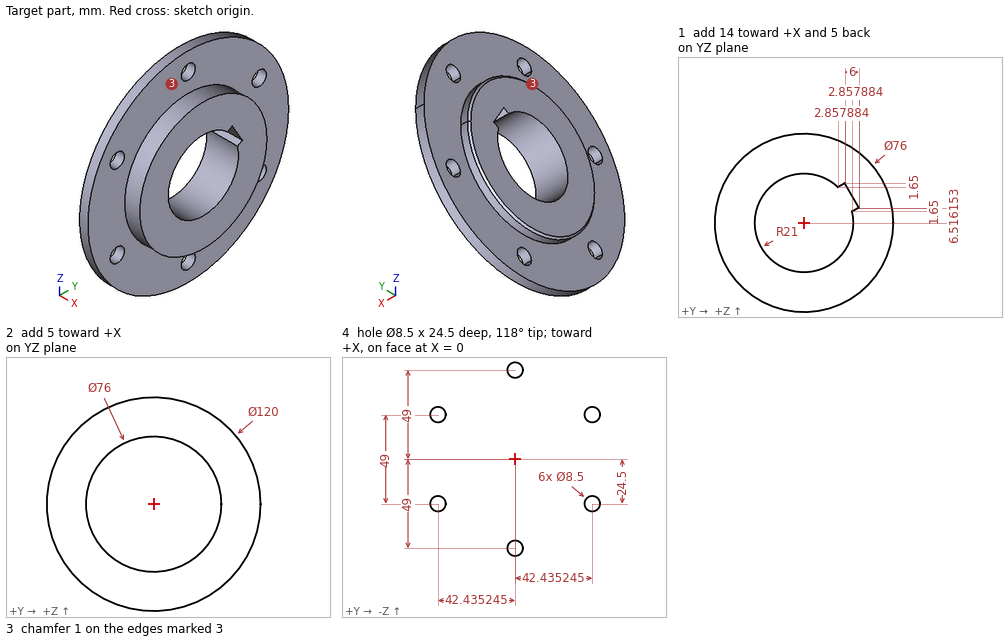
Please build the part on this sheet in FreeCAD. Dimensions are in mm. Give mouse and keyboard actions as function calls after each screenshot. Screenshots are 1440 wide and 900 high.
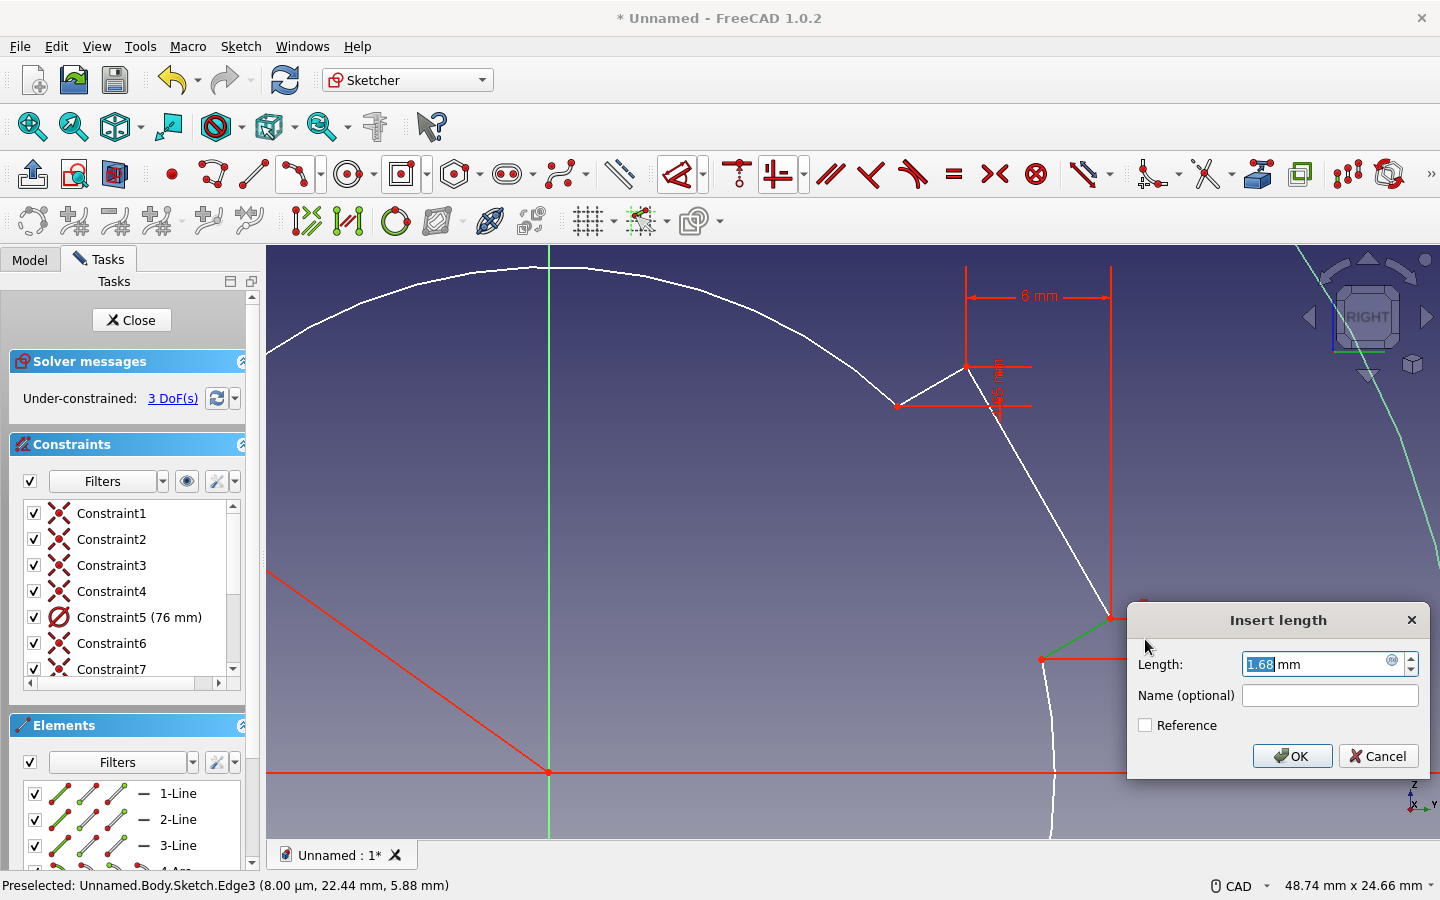
text(1.65)
key(Return)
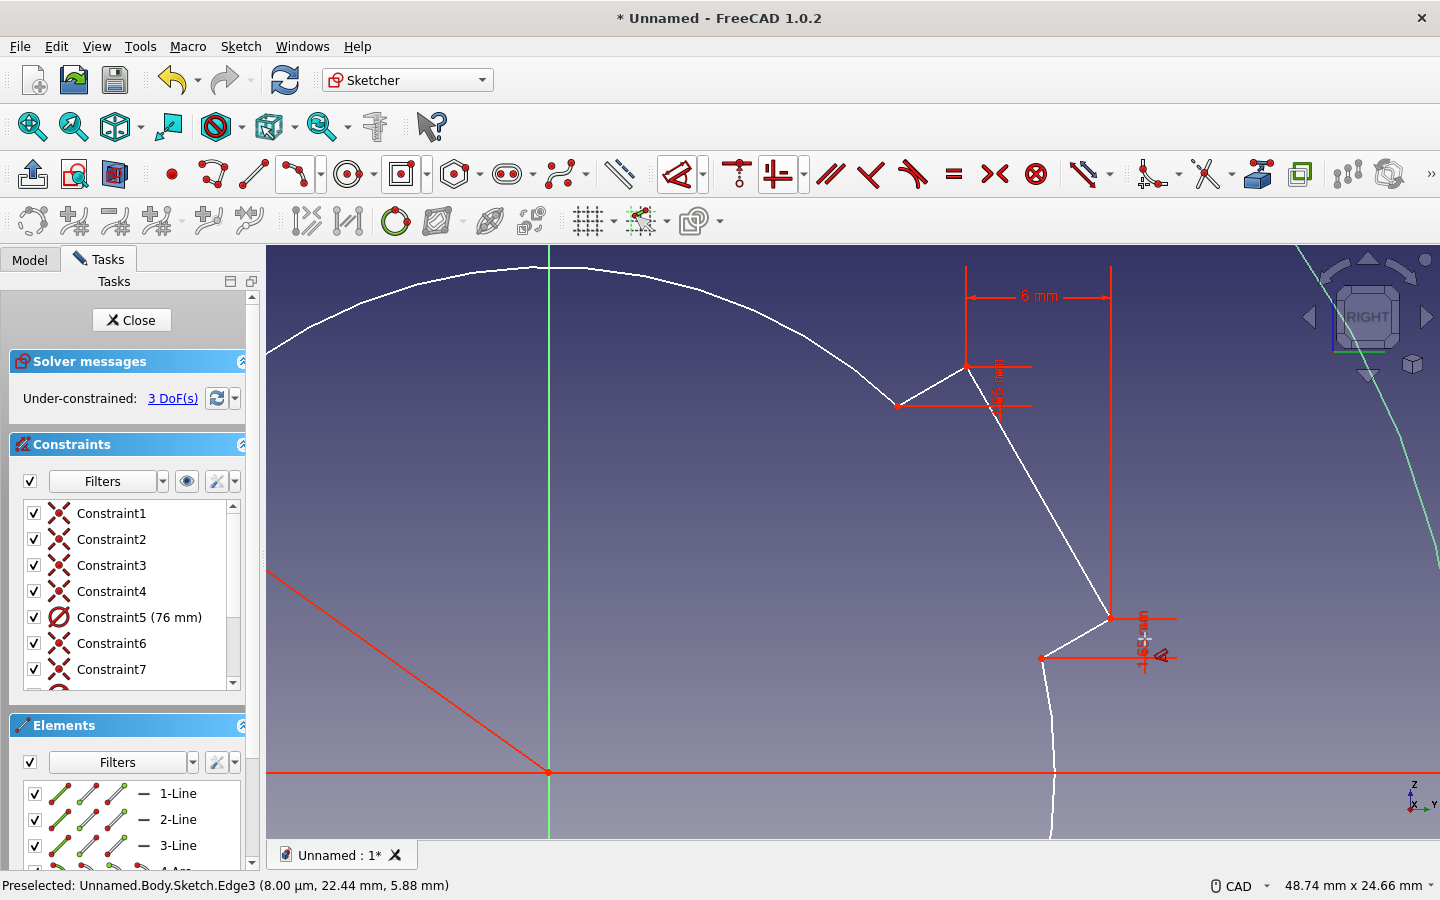
scroll(844, 484, down, 8)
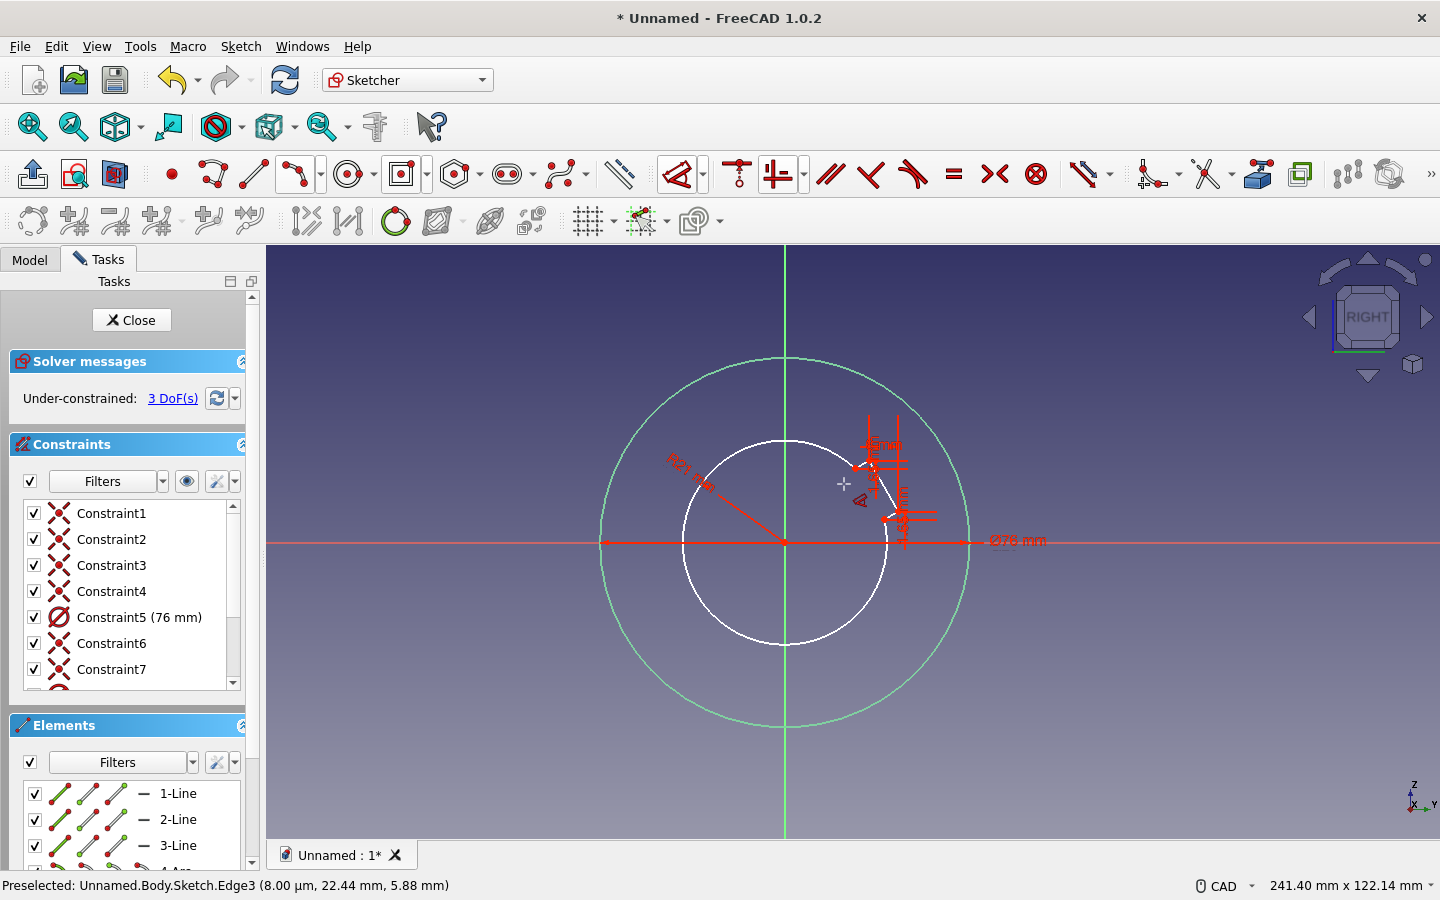
scroll(898, 512, up, 2)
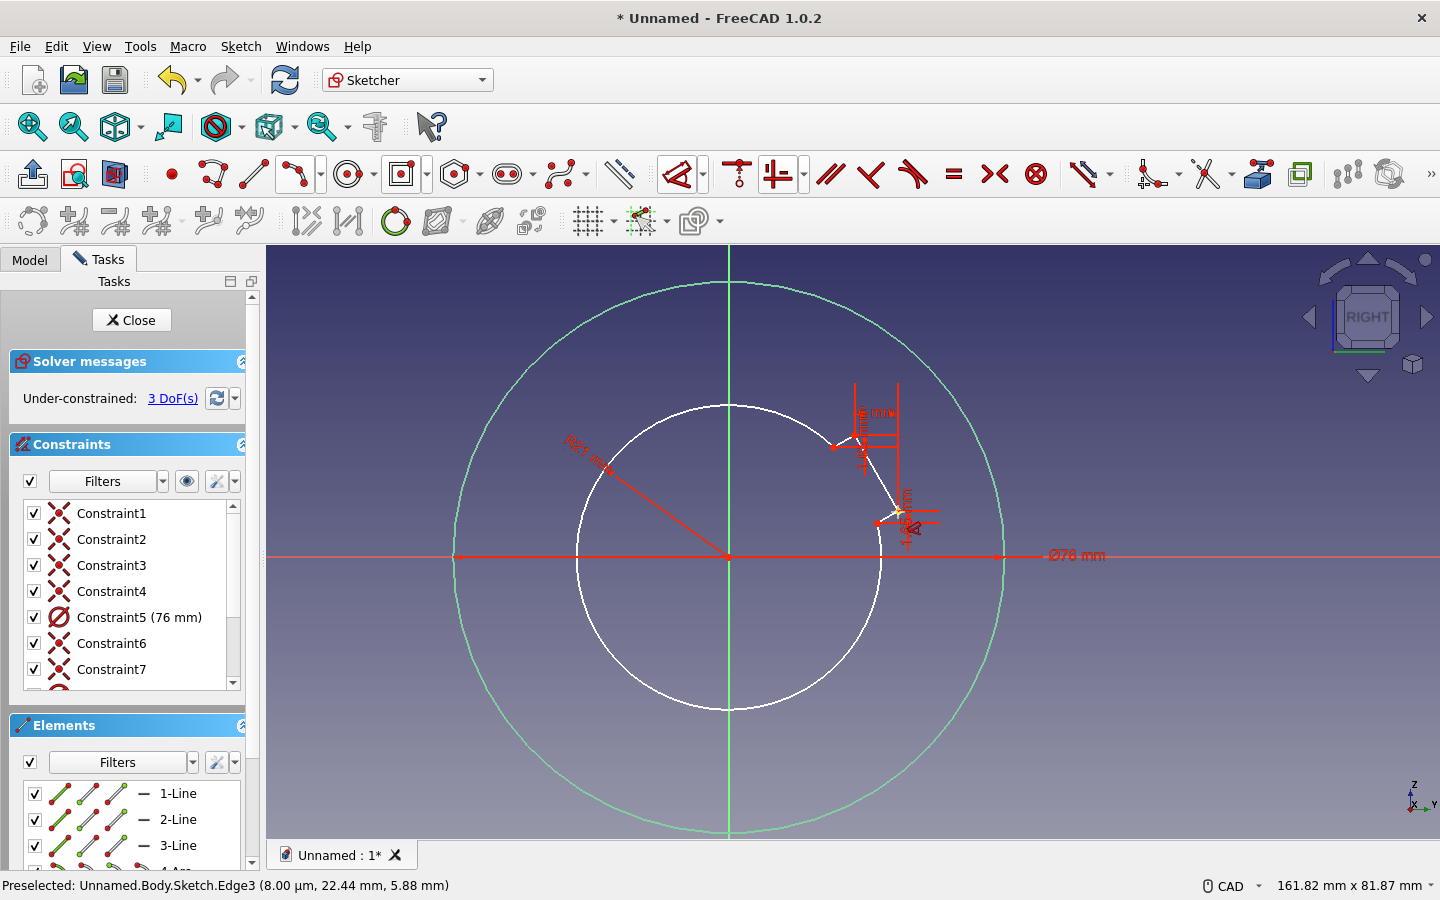
click(898, 511)
click(695, 534)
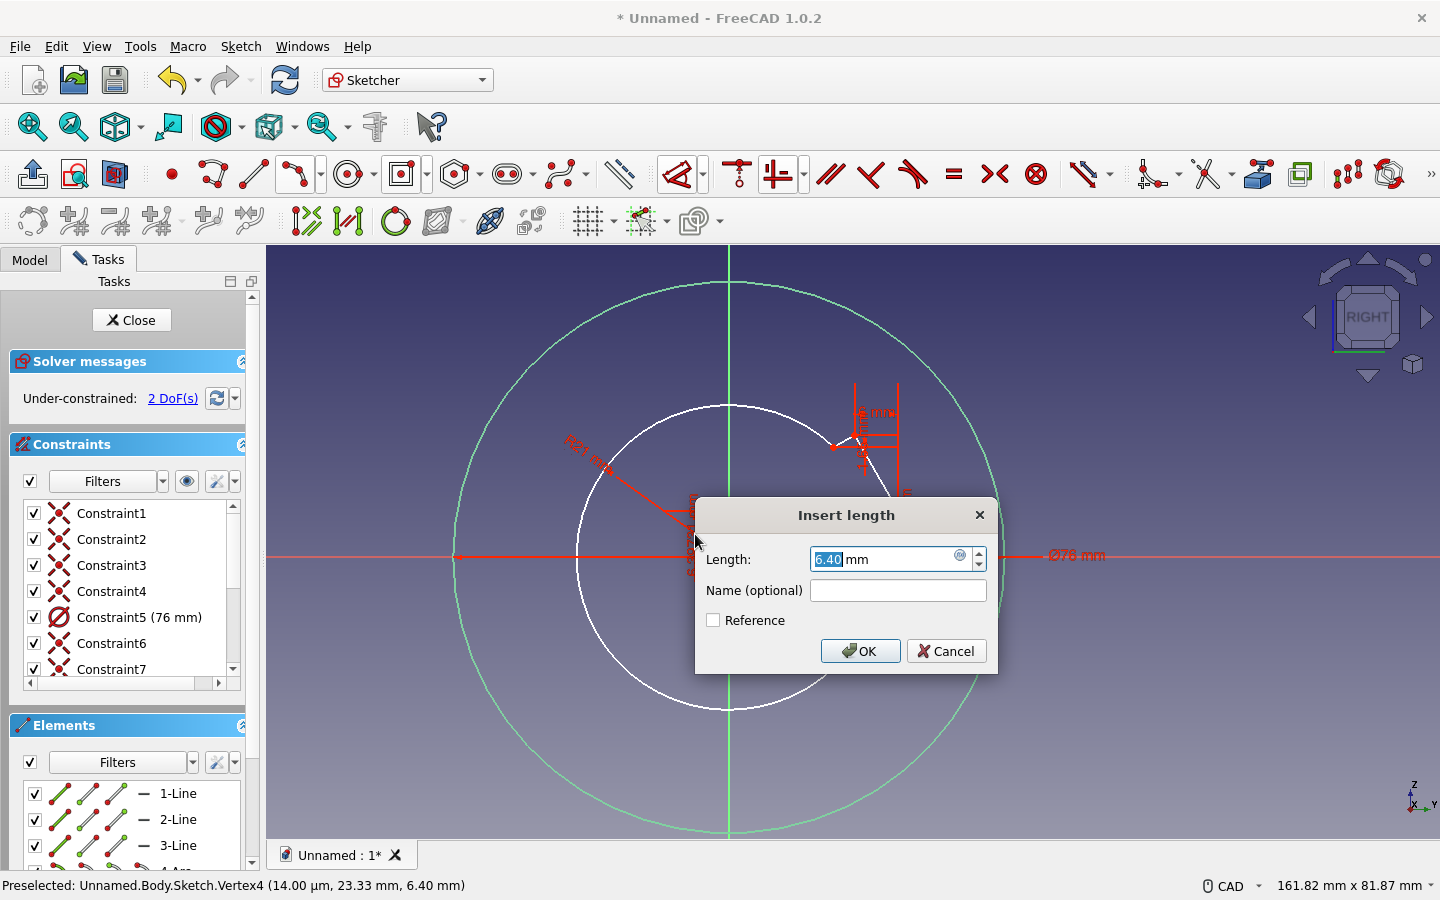
text(6.516153)
key(Return)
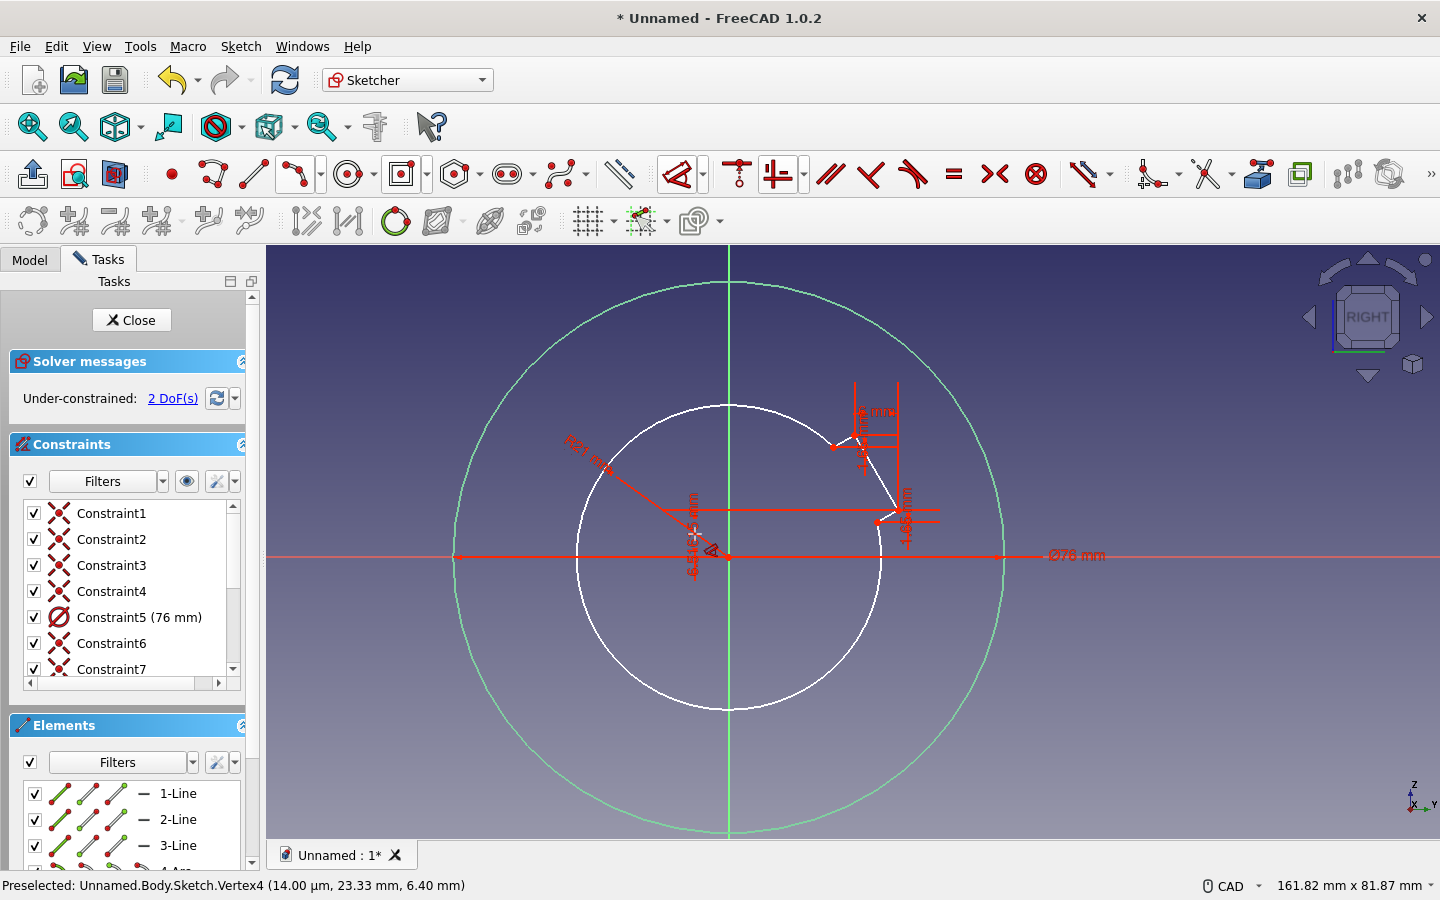
scroll(842, 442, up, 4)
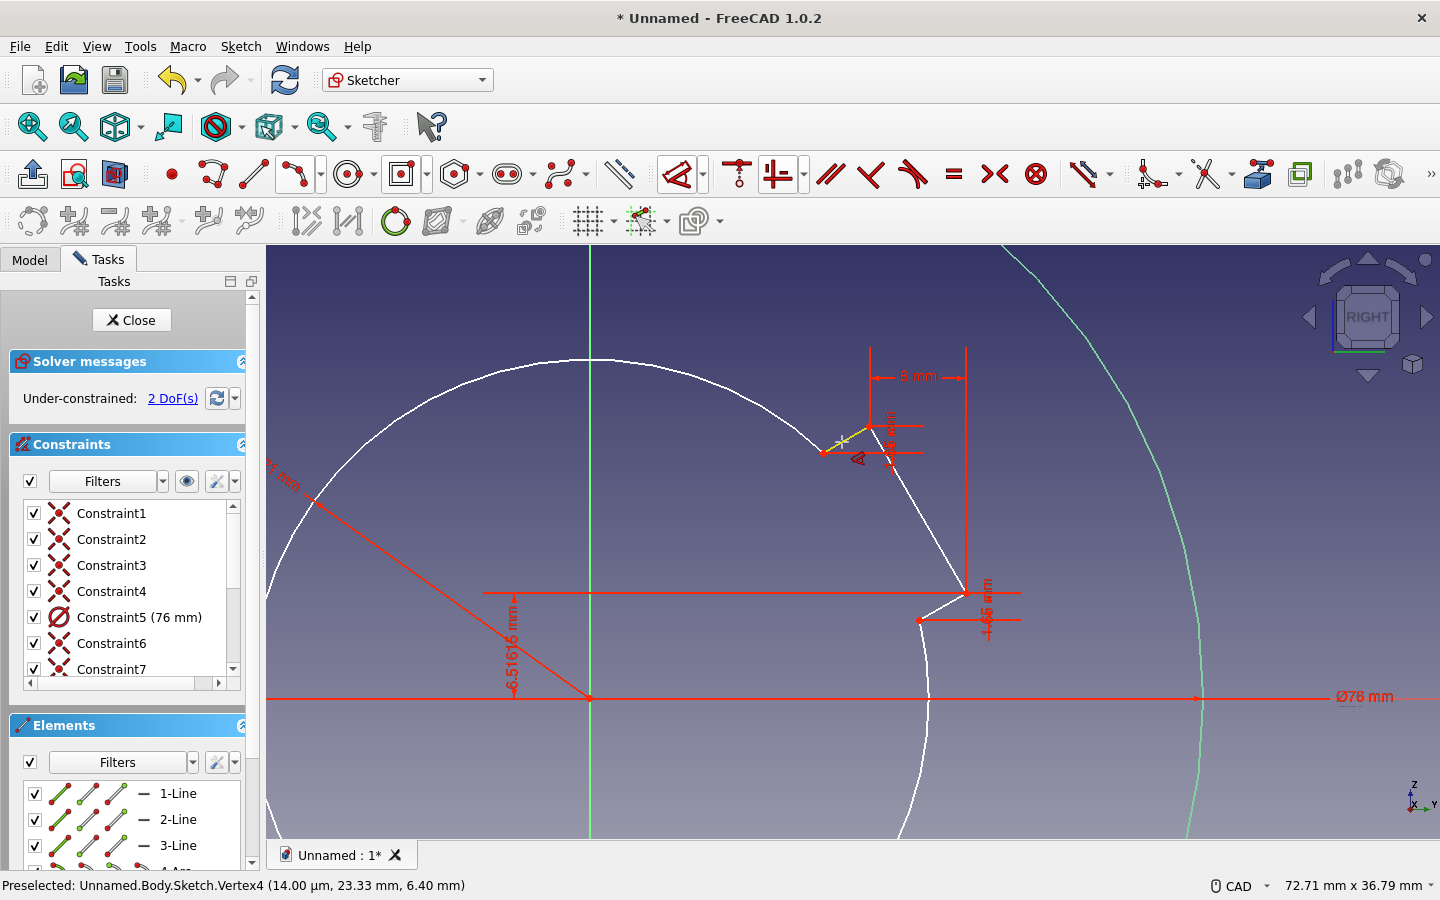
click(842, 442)
click(846, 392)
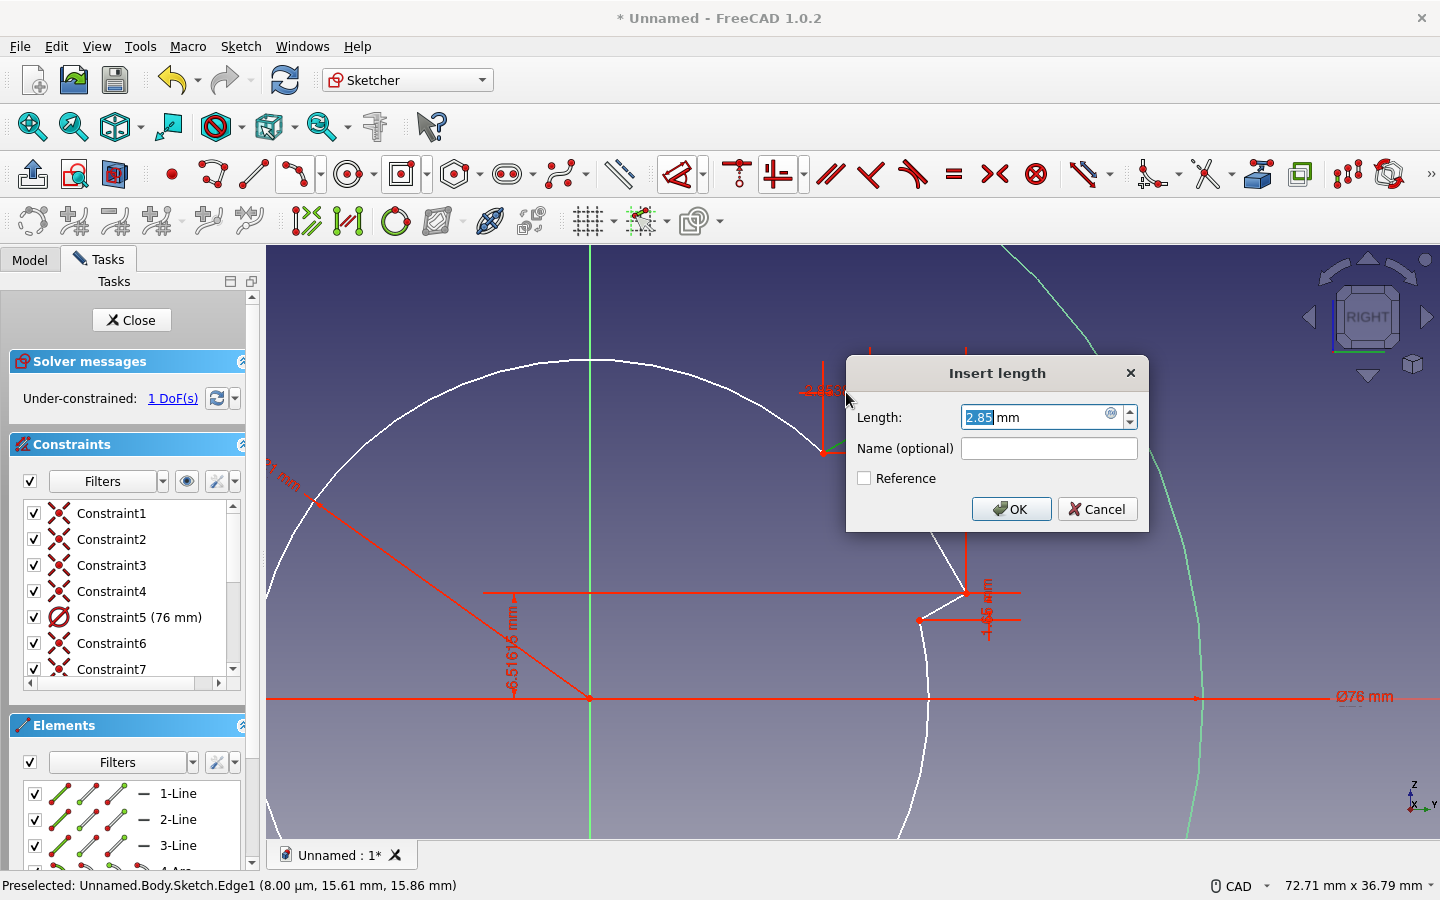
text(2.857884)
key(Return)